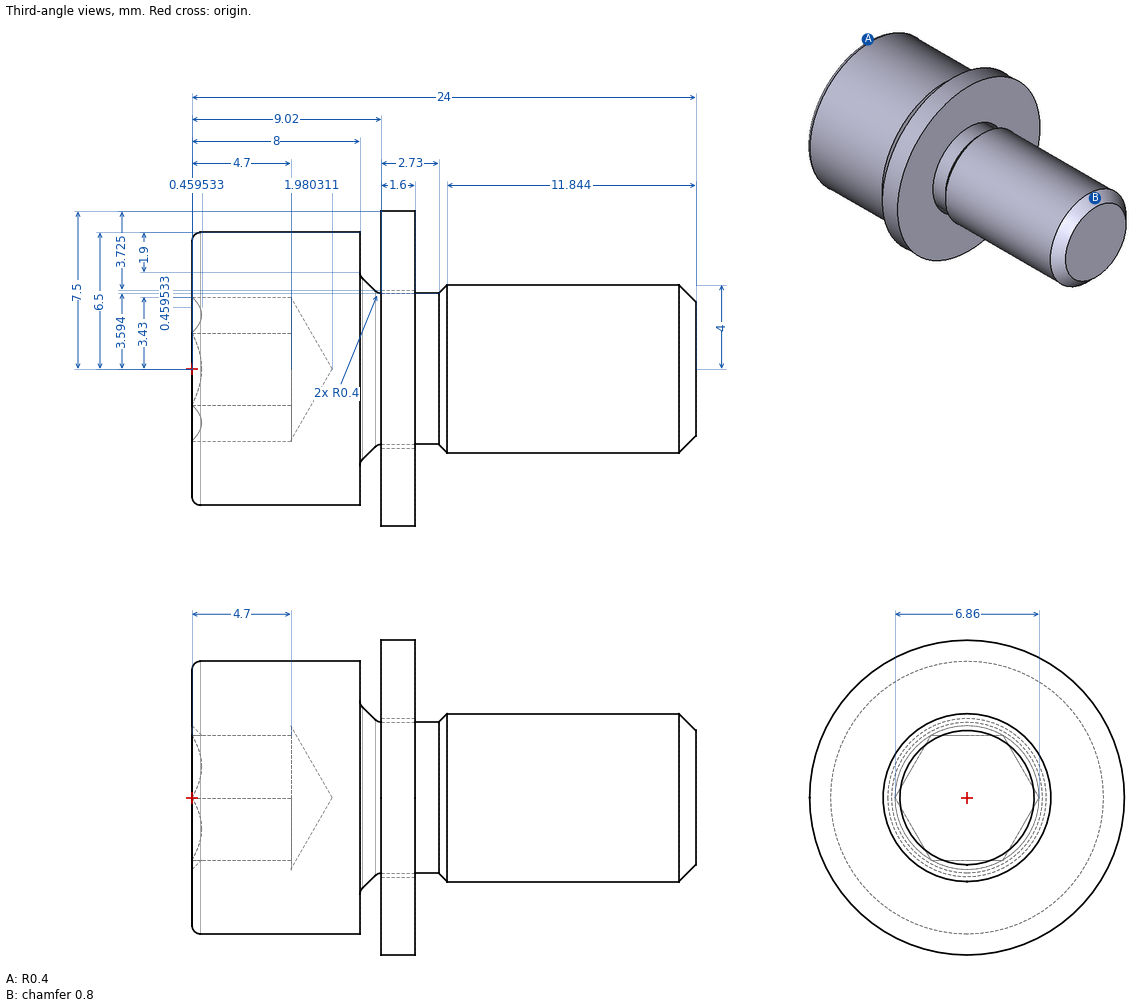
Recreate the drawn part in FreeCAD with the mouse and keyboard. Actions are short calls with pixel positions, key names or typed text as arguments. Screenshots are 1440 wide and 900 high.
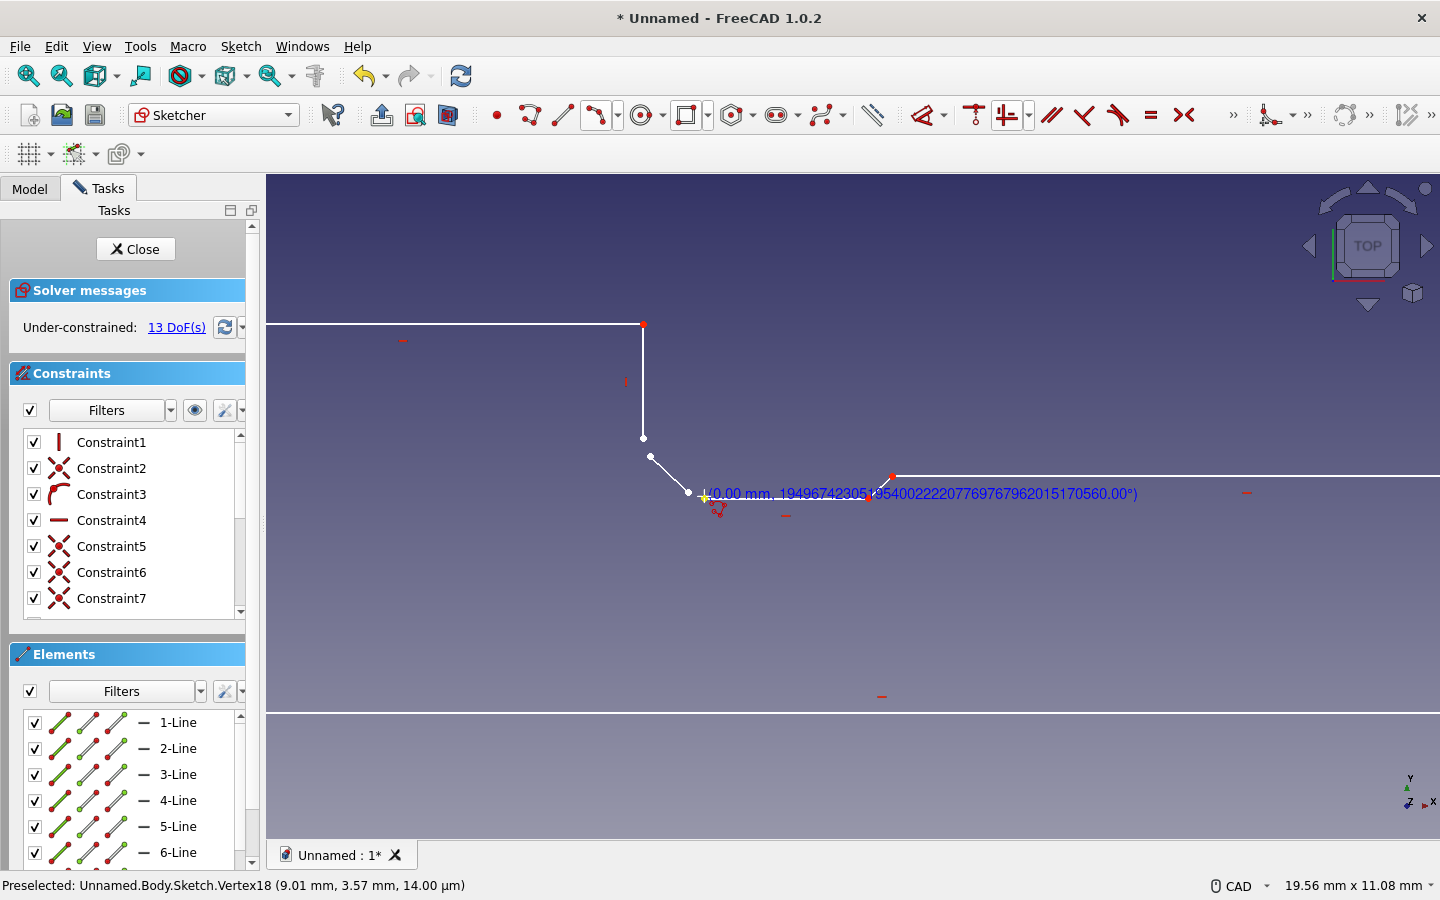
click(596, 116)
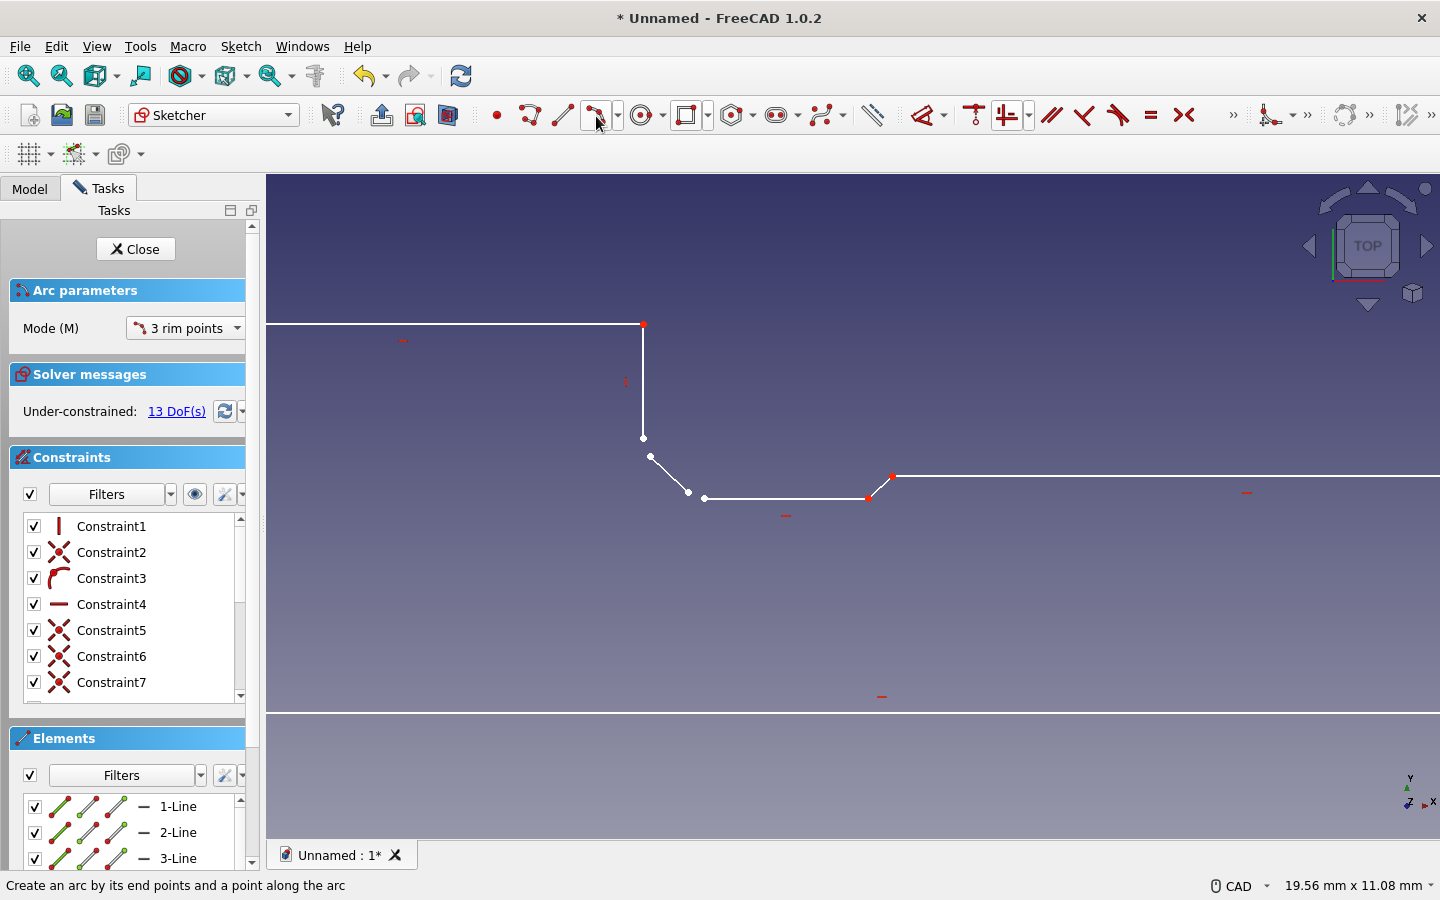
click(650, 457)
click(643, 438)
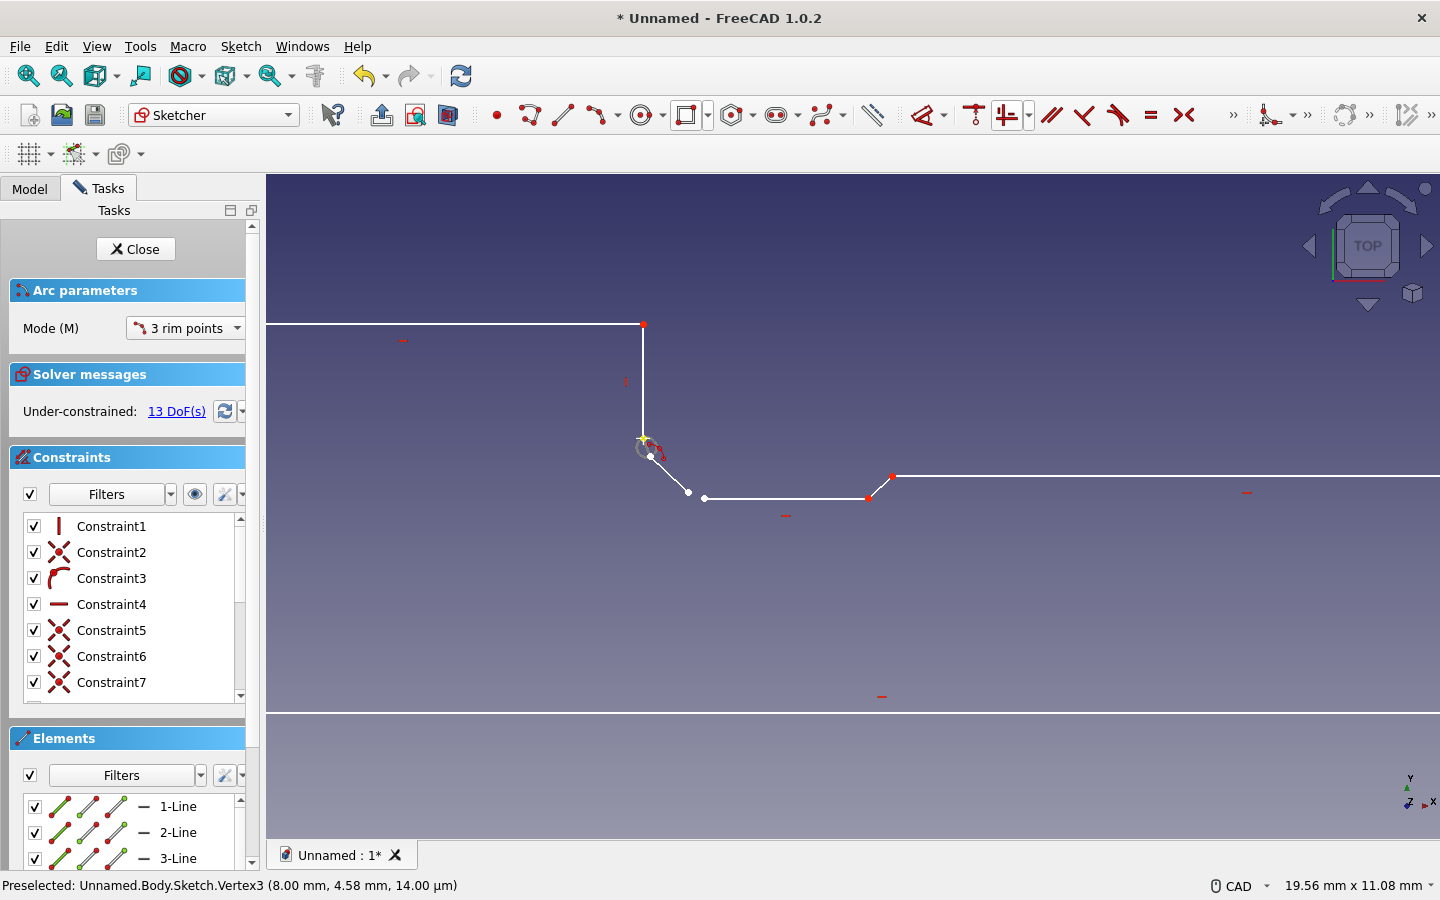
scroll(645, 446, up, 11)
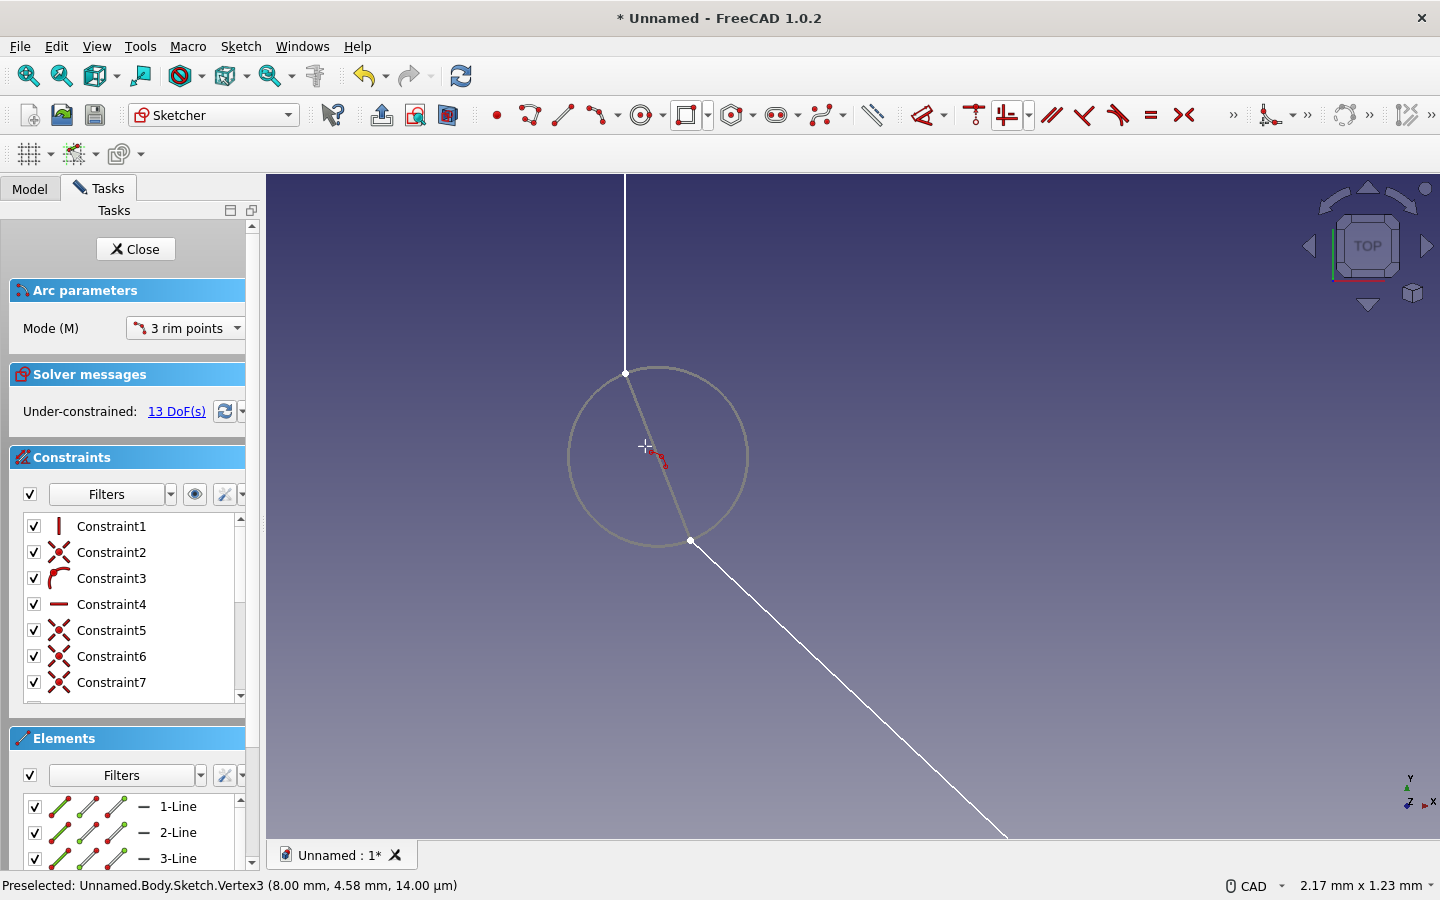
click(644, 446)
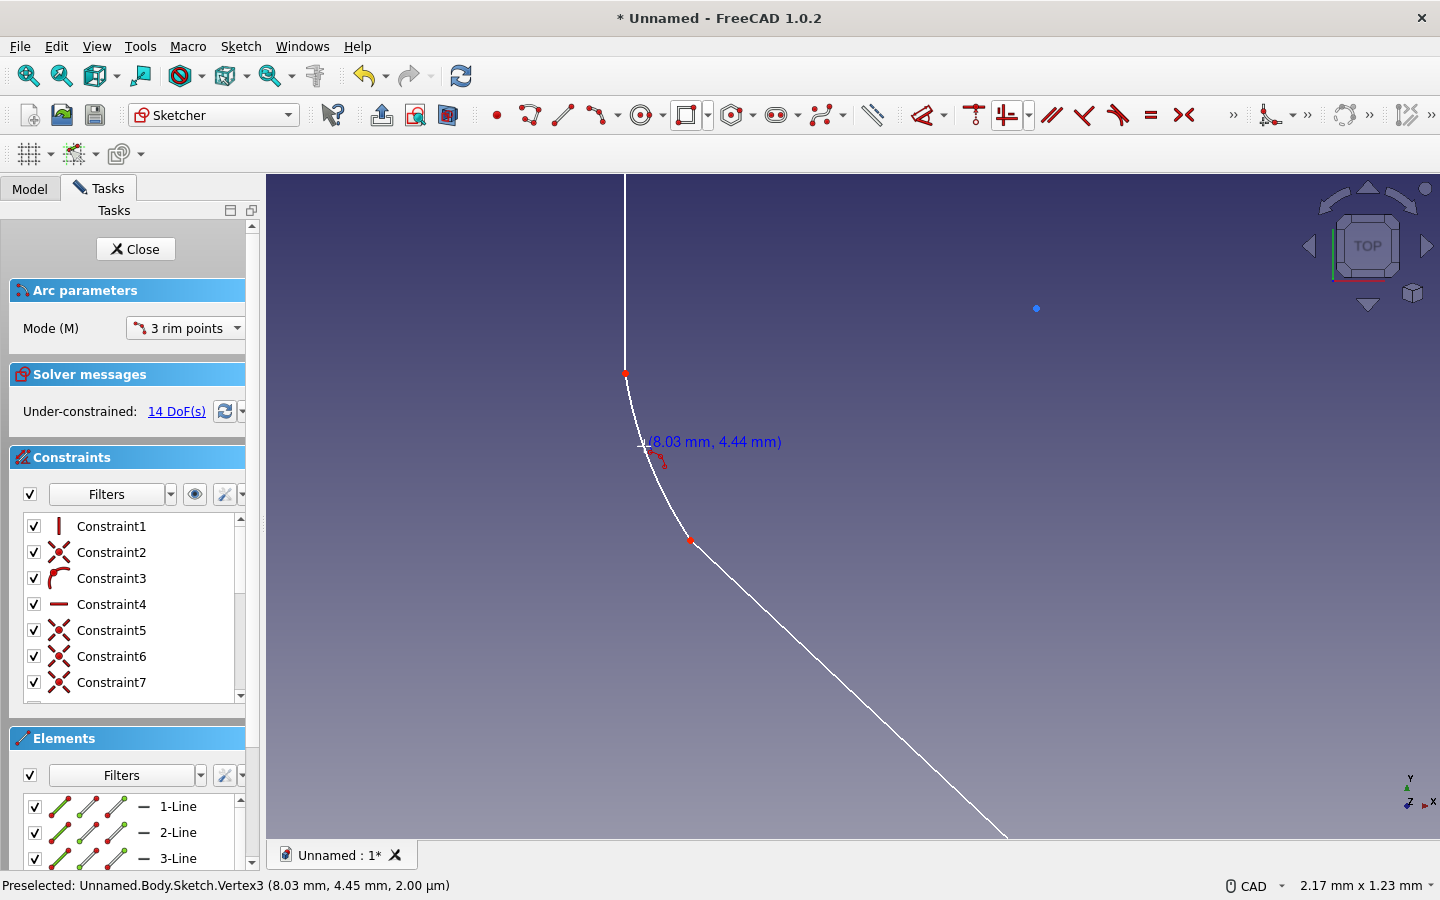
scroll(679, 476, down, 15)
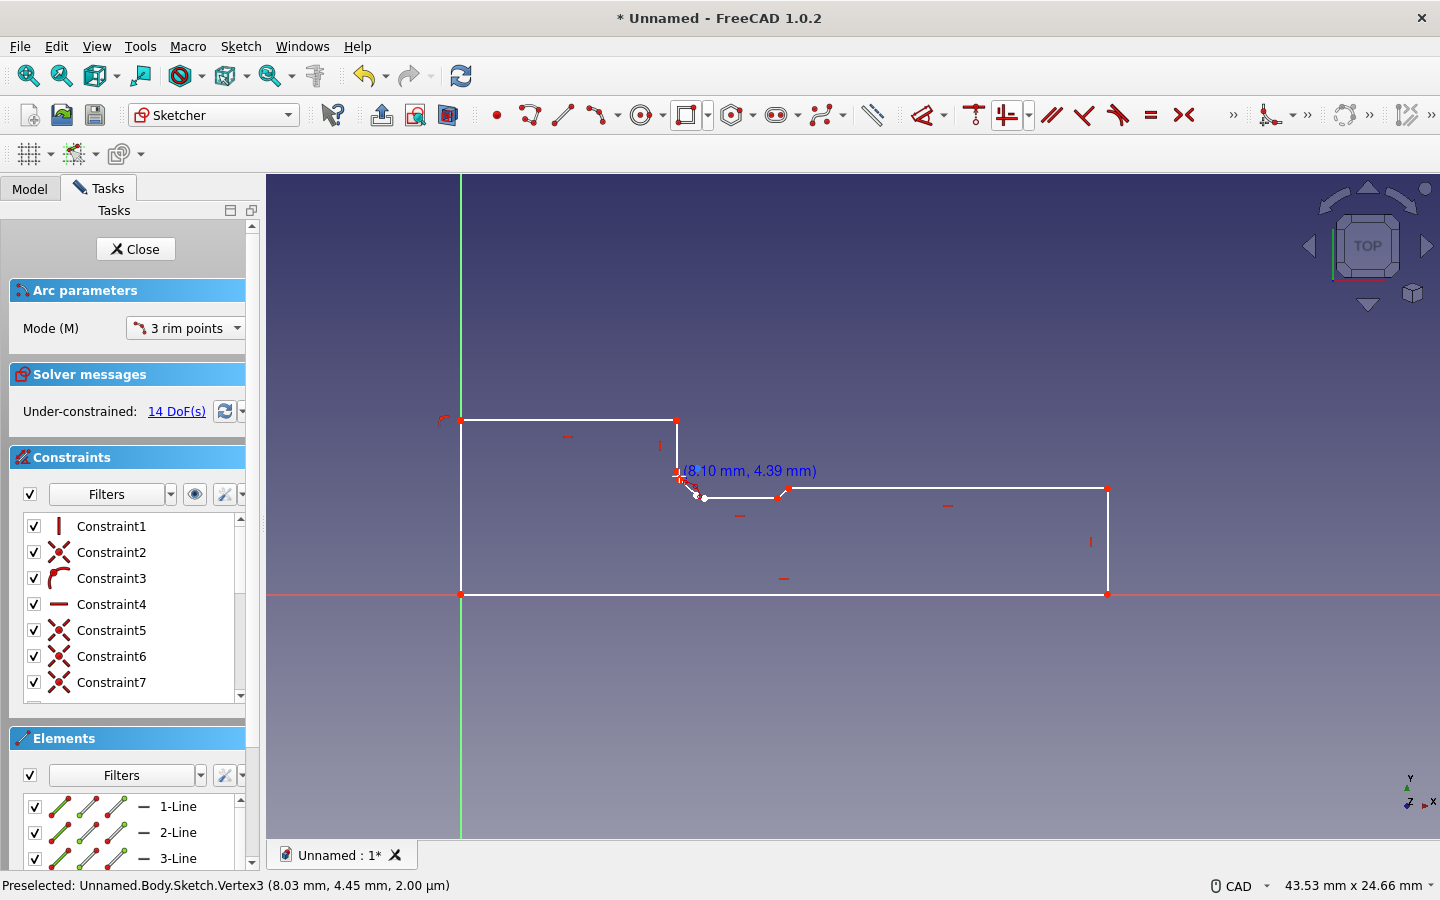
scroll(704, 498, up, 4)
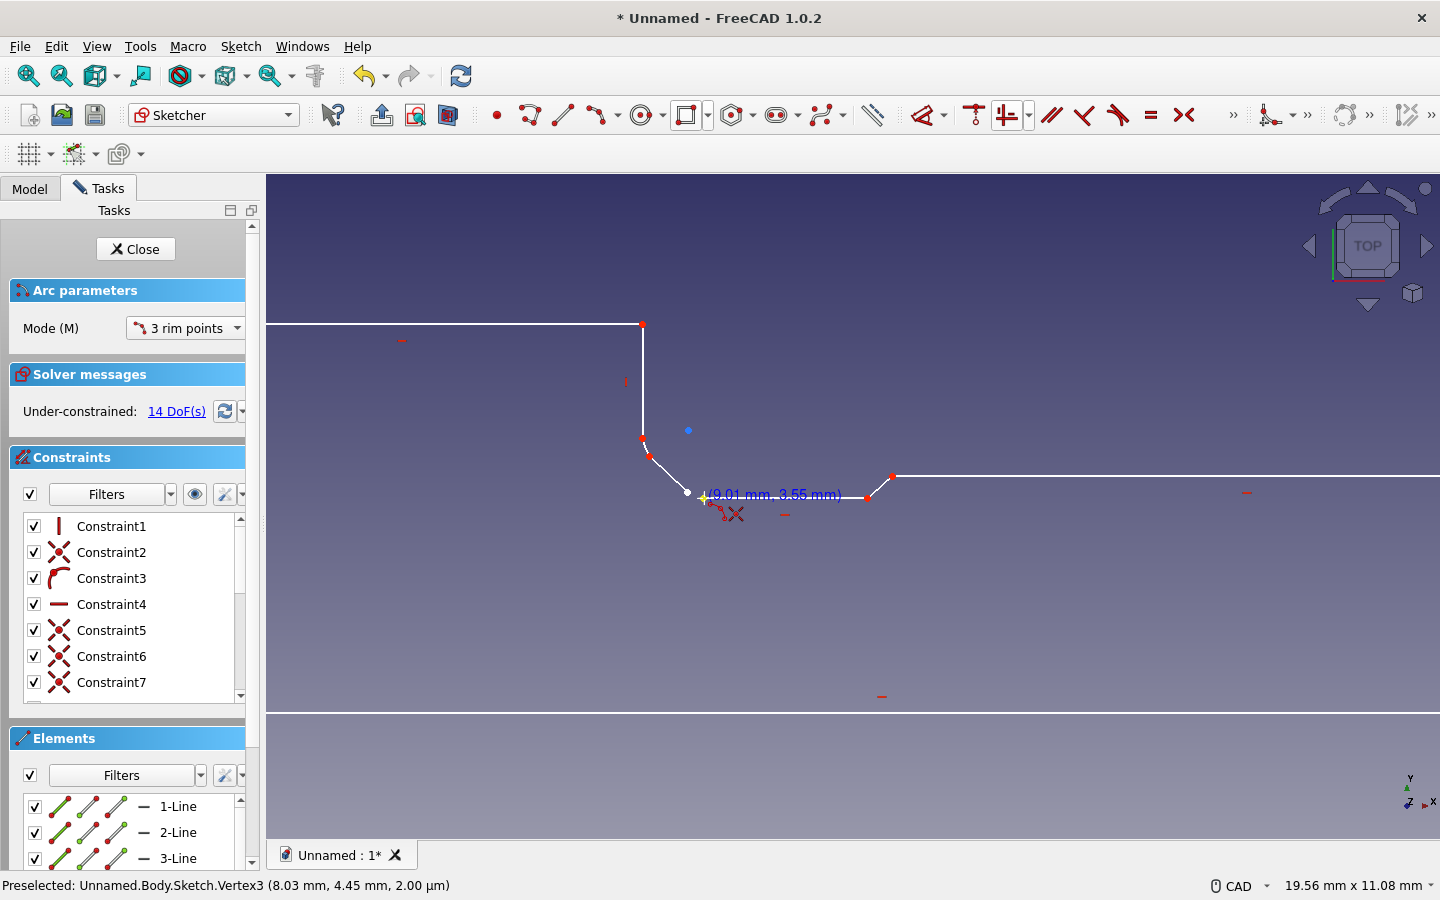
click(704, 498)
click(688, 492)